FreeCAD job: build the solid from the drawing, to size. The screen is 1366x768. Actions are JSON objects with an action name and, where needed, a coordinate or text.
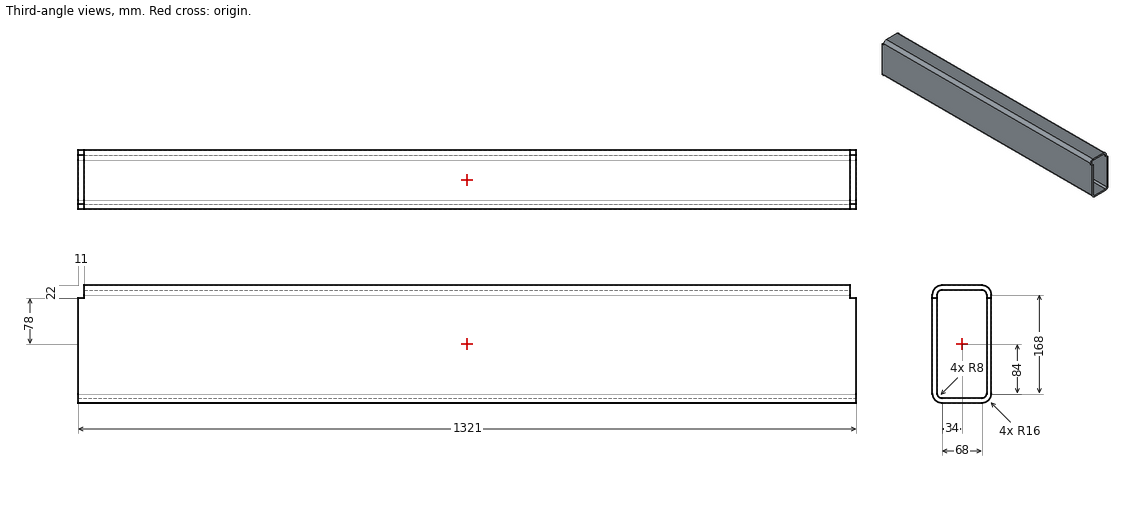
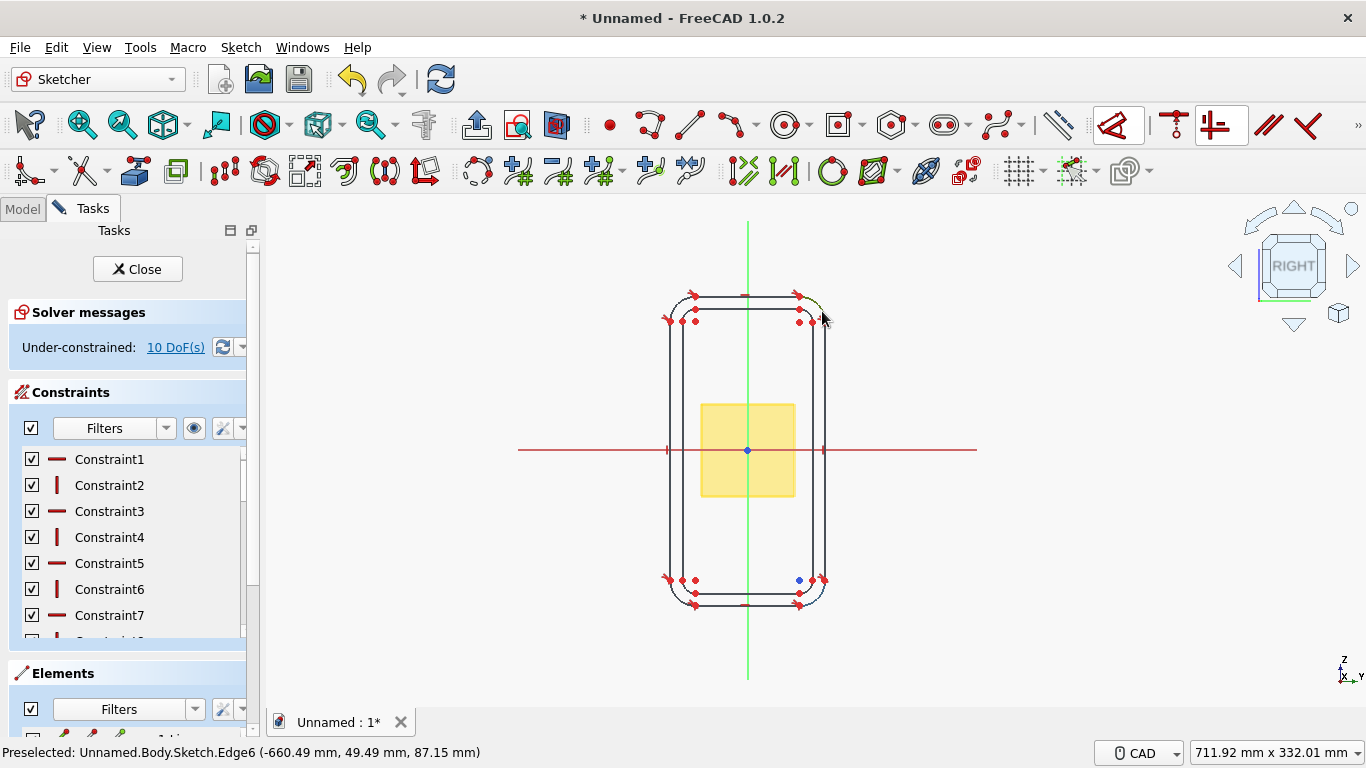
{"action": "left_click", "coordinate": [684, 300]}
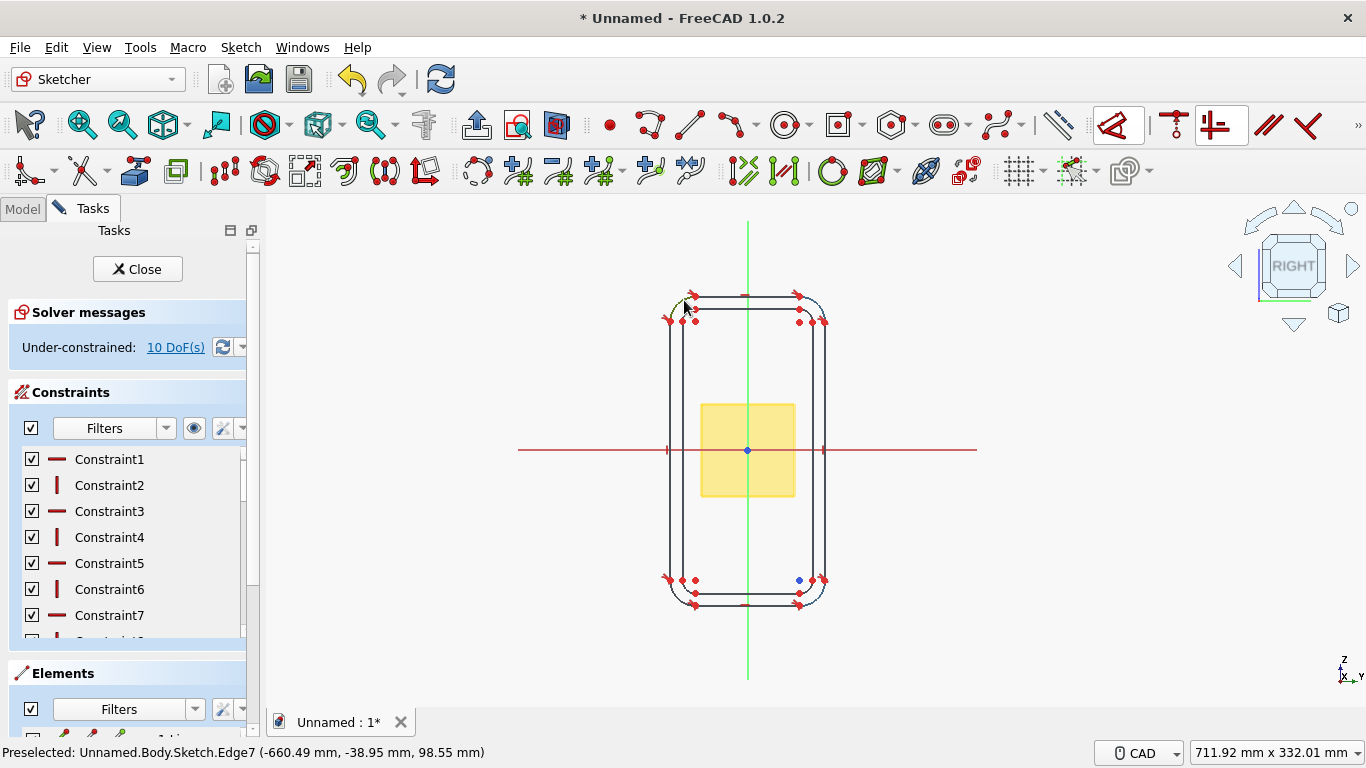
{"action": "left_click", "coordinate": [673, 592]}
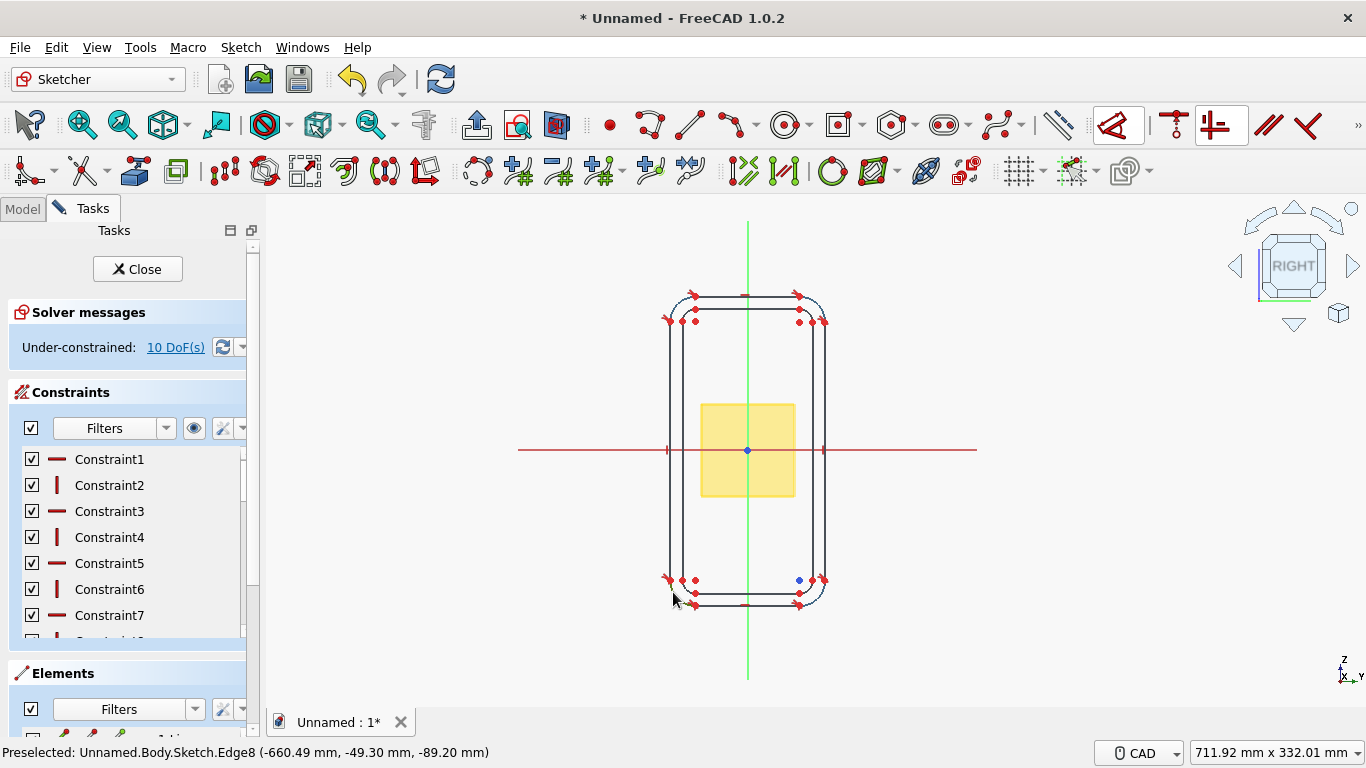
{"action": "key", "text": "e"}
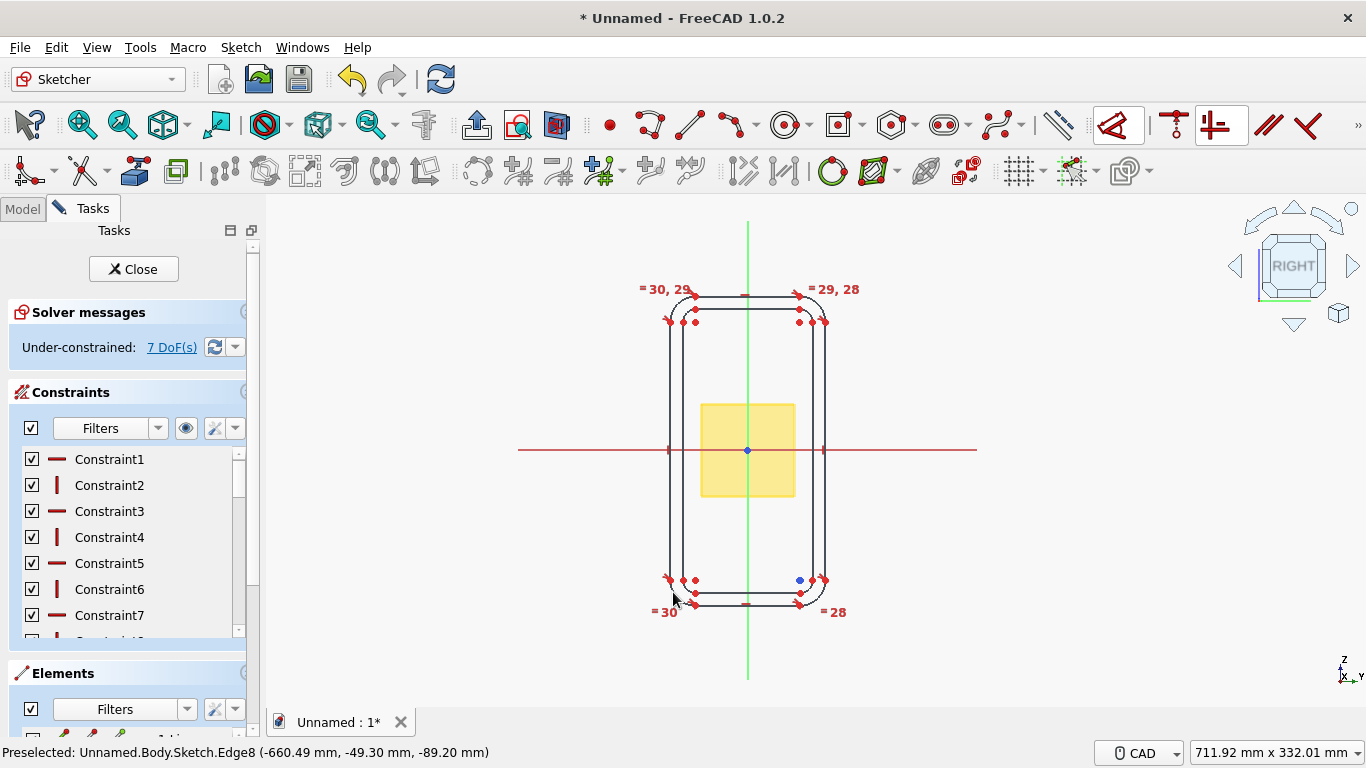
{"action": "scroll", "coordinate": [687, 589], "scroll_direction": "up", "scroll_amount": 2}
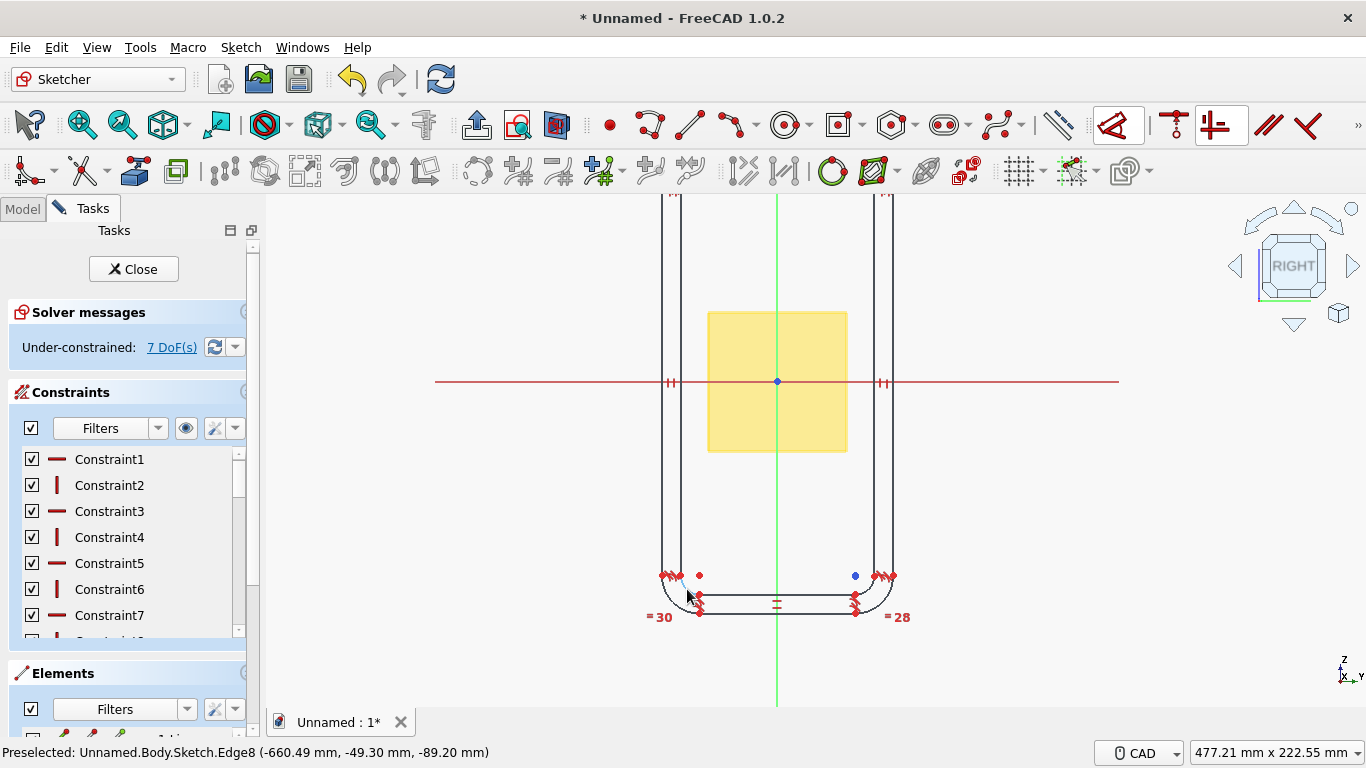
{"action": "left_click", "coordinate": [687, 589]}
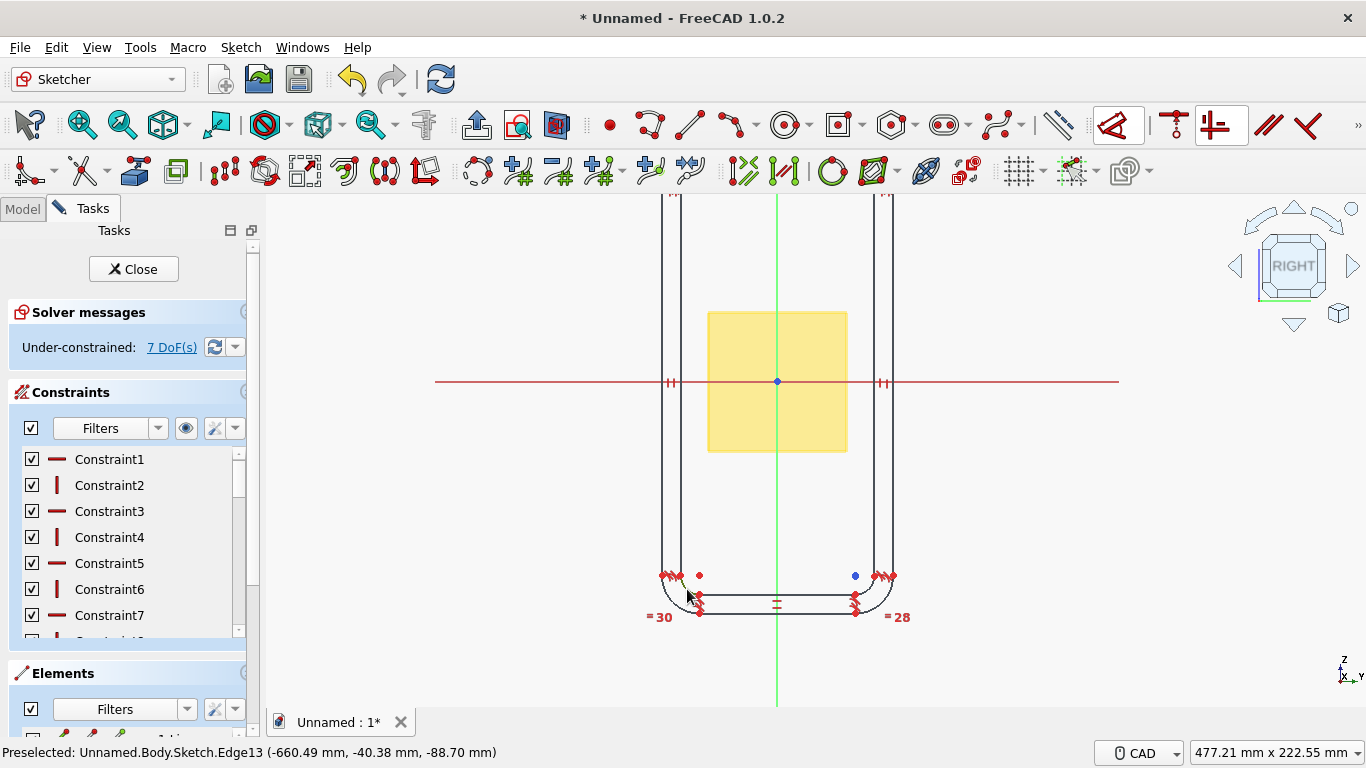
{"action": "left_click", "coordinate": [869, 589]}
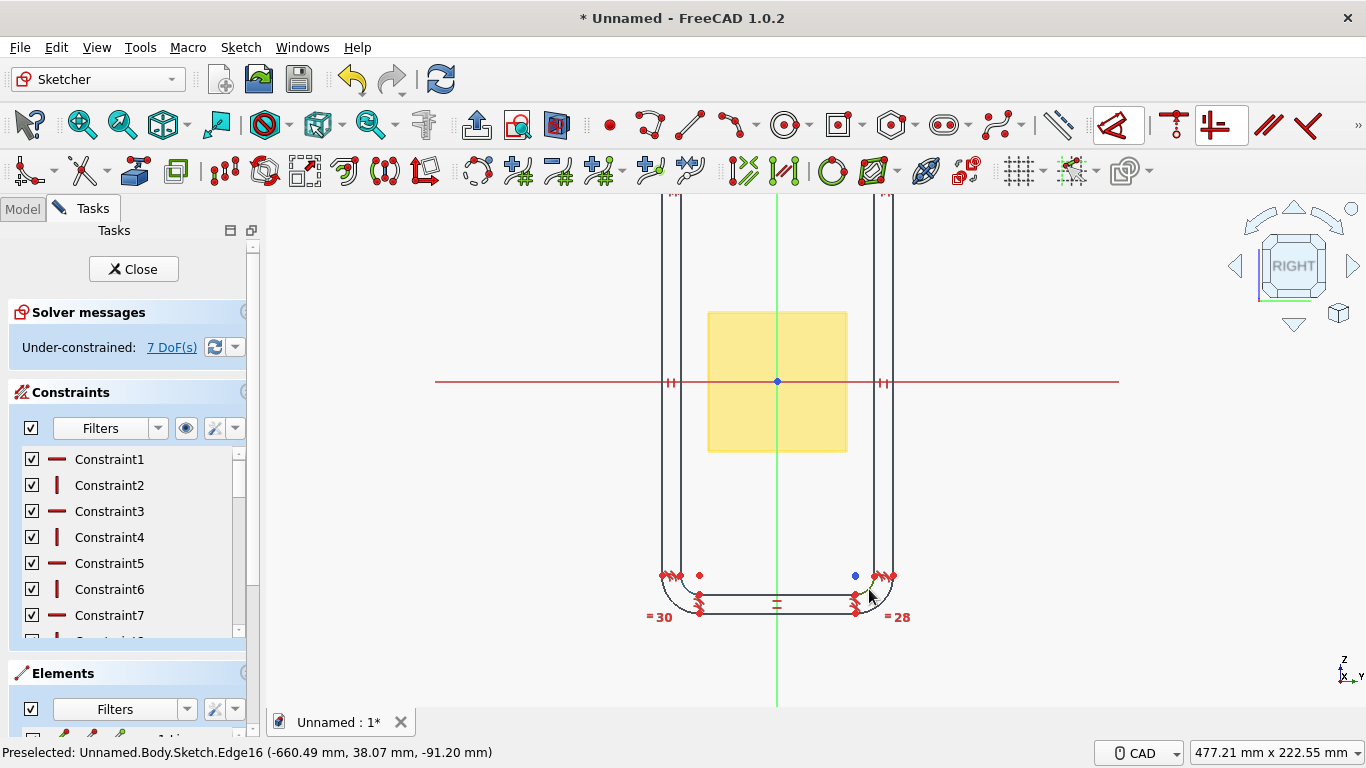
{"action": "key", "text": "e"}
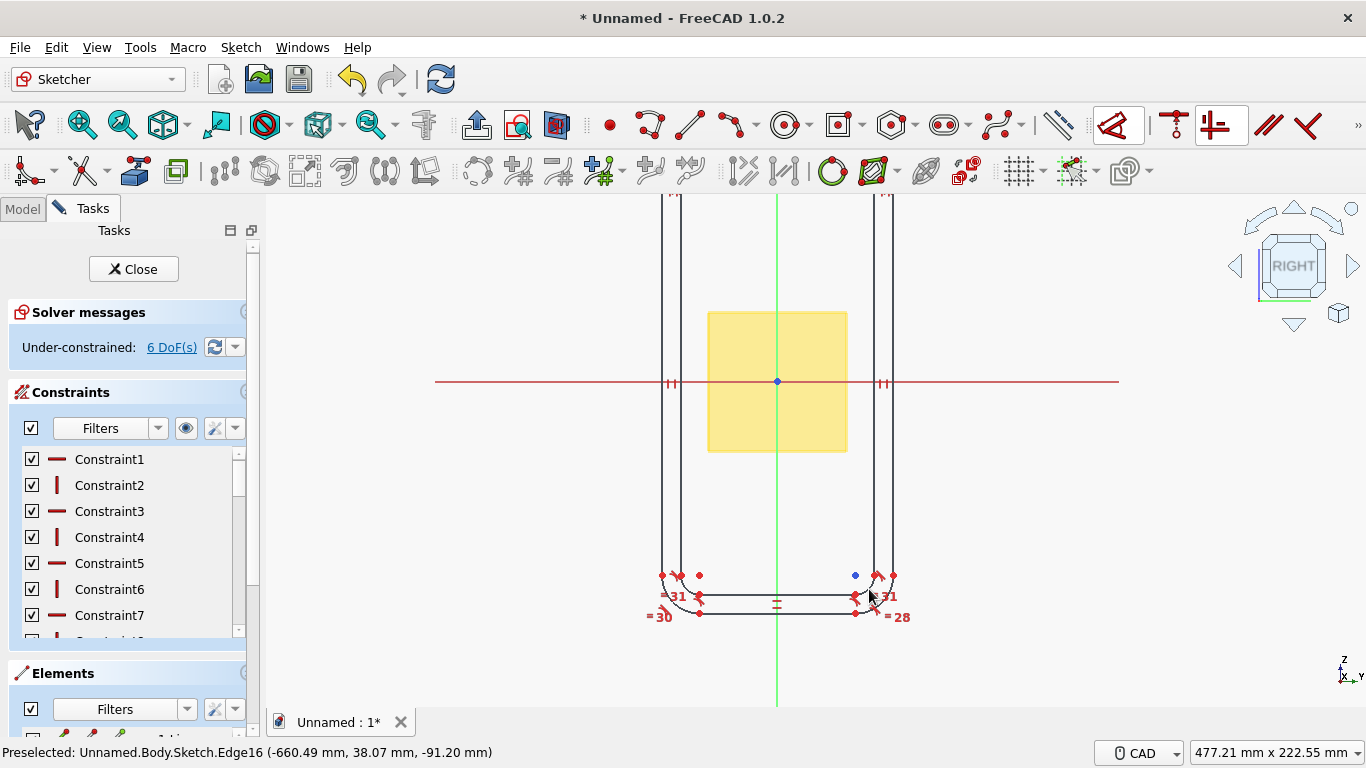
{"action": "left_click", "coordinate": [1112, 126]}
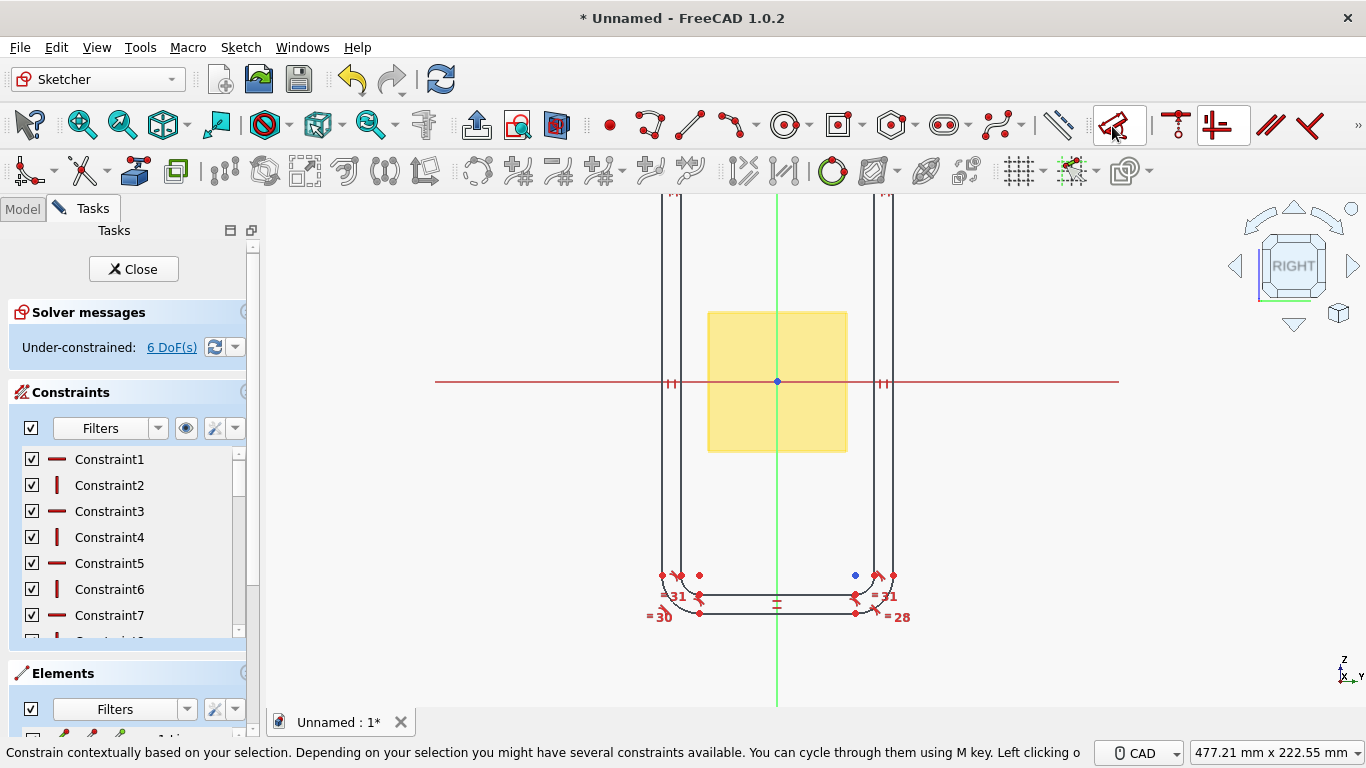
{"action": "left_click", "coordinate": [872, 610]}
{"action": "left_click", "coordinate": [886, 639]}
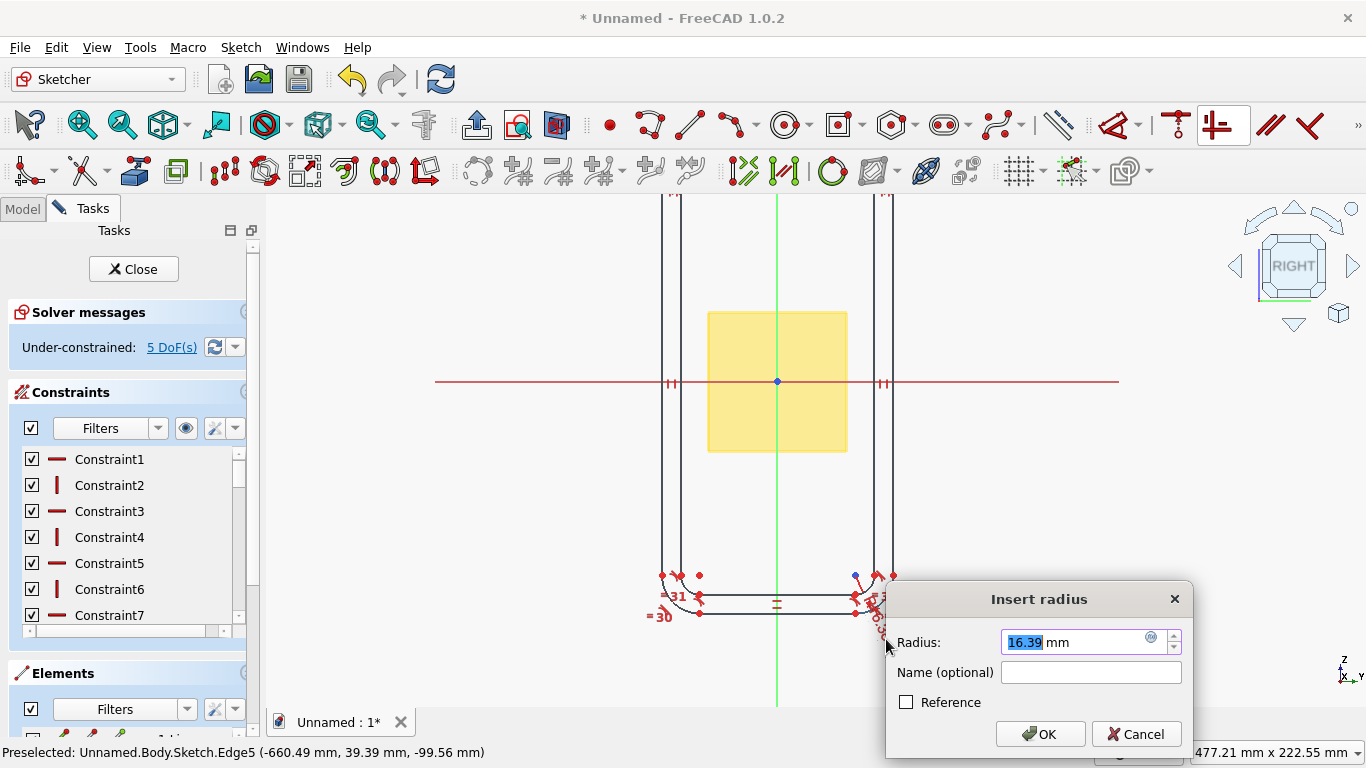
{"action": "type", "text": "16"}
{"action": "key", "text": "Return"}